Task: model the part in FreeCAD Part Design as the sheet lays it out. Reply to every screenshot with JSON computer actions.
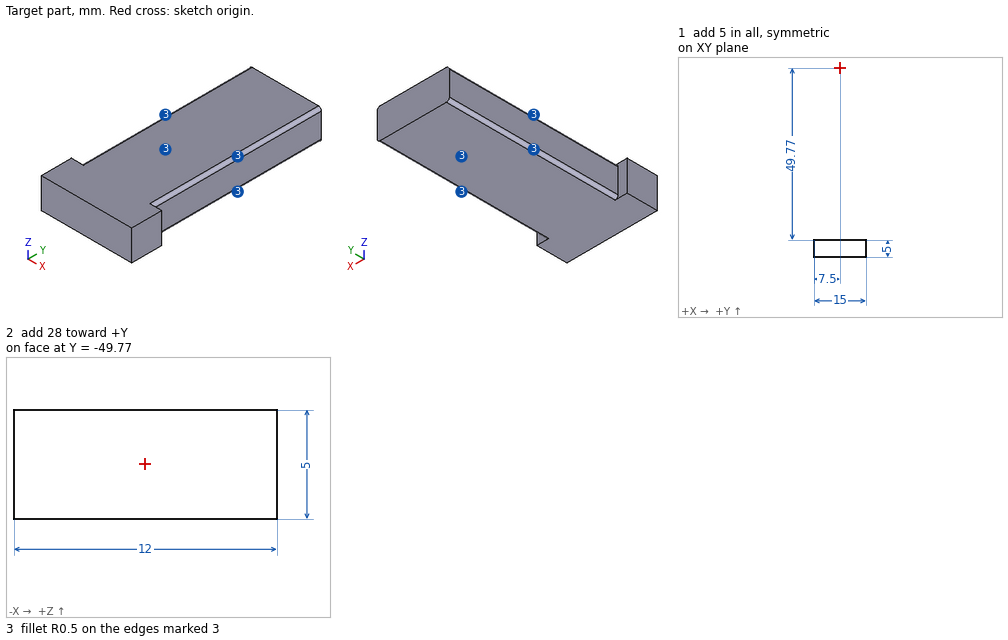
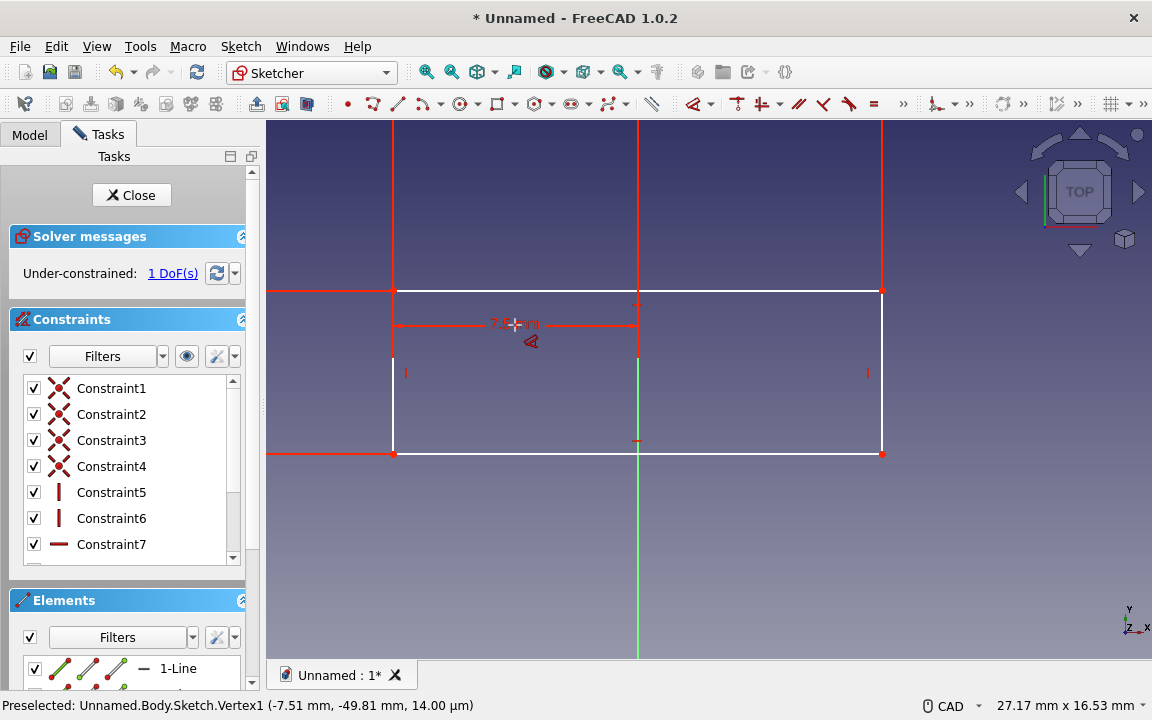
{"action": "left_click", "coordinate": [393, 291]}
{"action": "left_click", "coordinate": [359, 220]}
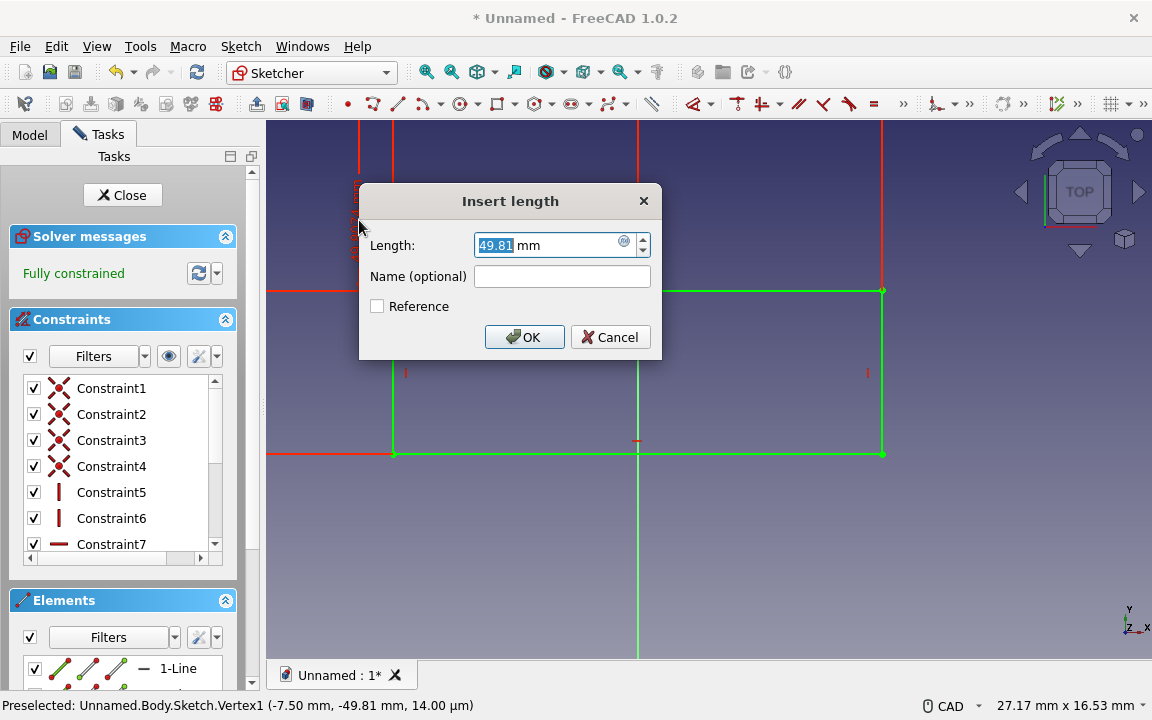
{"action": "type", "text": "49.77"}
{"action": "key", "text": "Return"}
{"action": "key", "text": "Escape"}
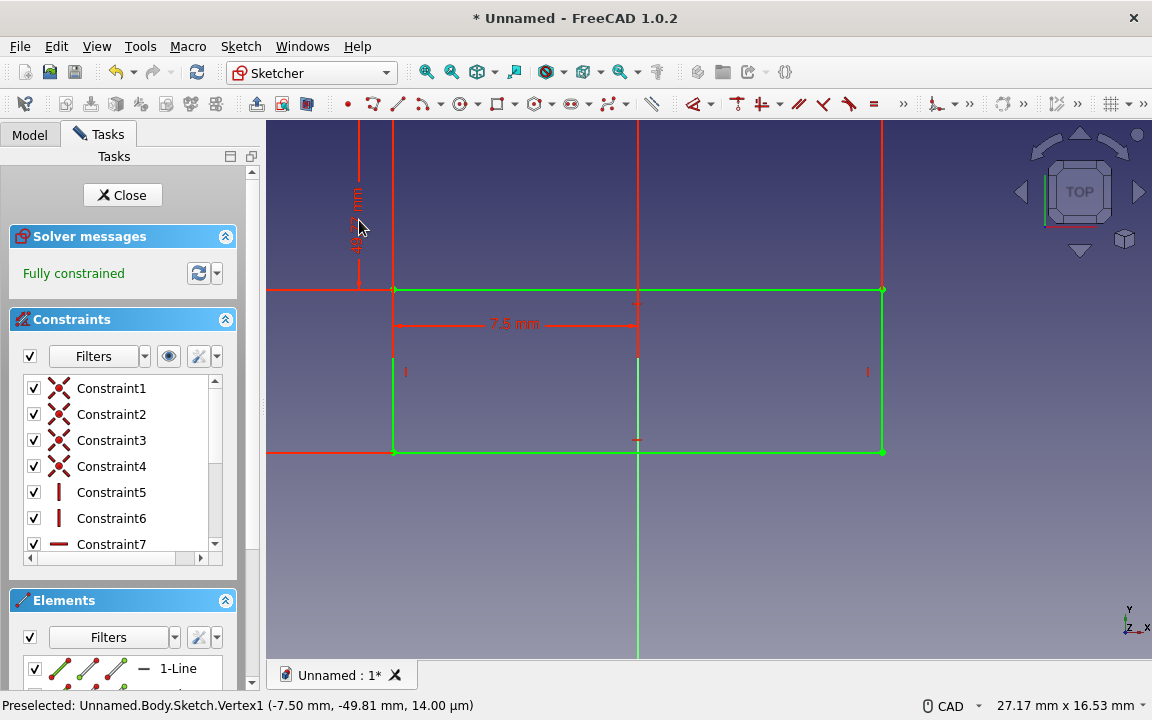
{"action": "left_click", "coordinate": [123, 195]}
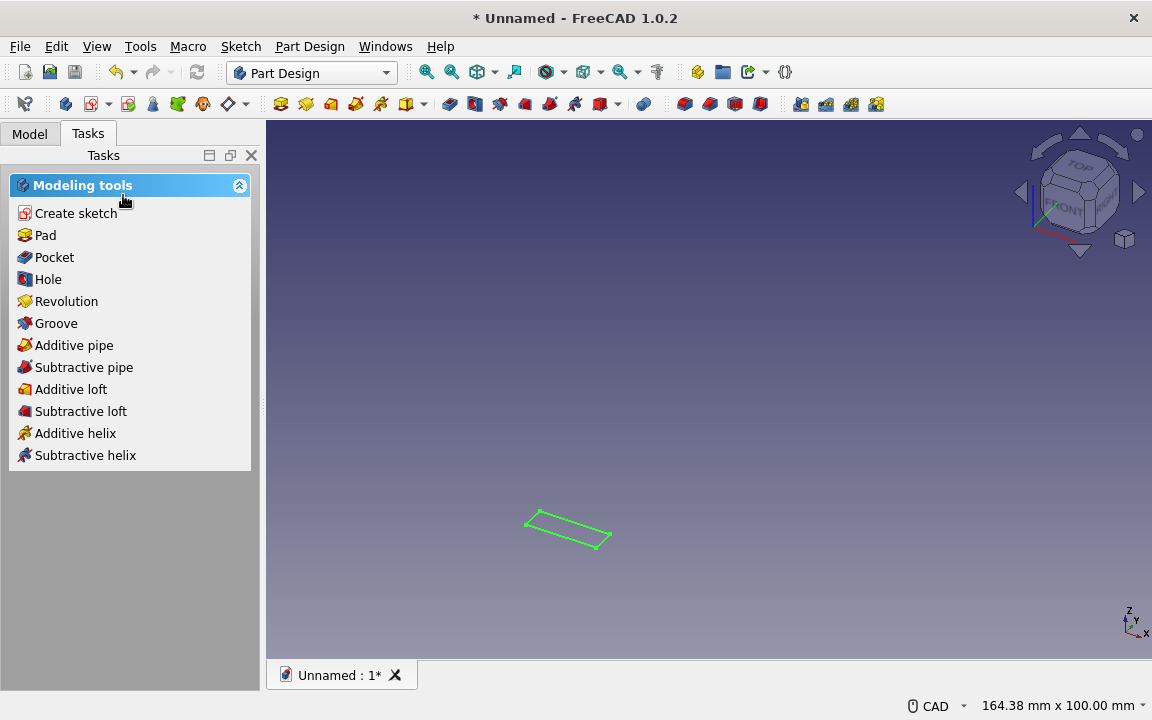
{"action": "left_click", "coordinate": [281, 104]}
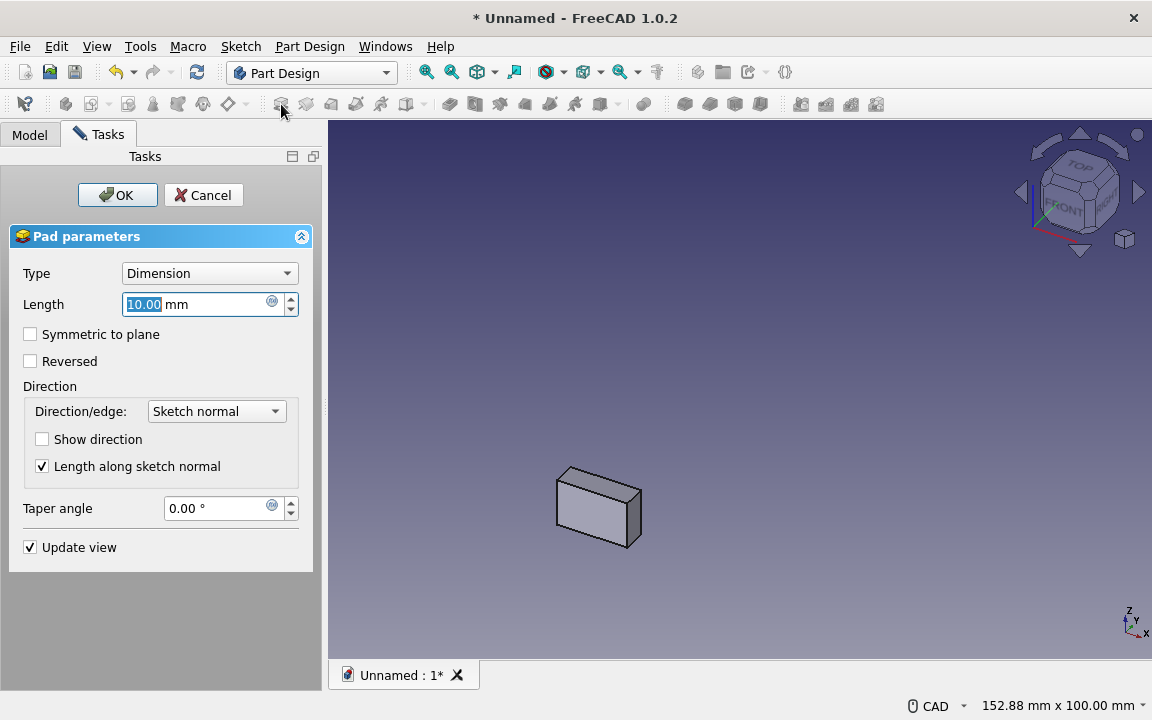
{"action": "type", "text": "5"}
{"action": "key", "text": "Tab"}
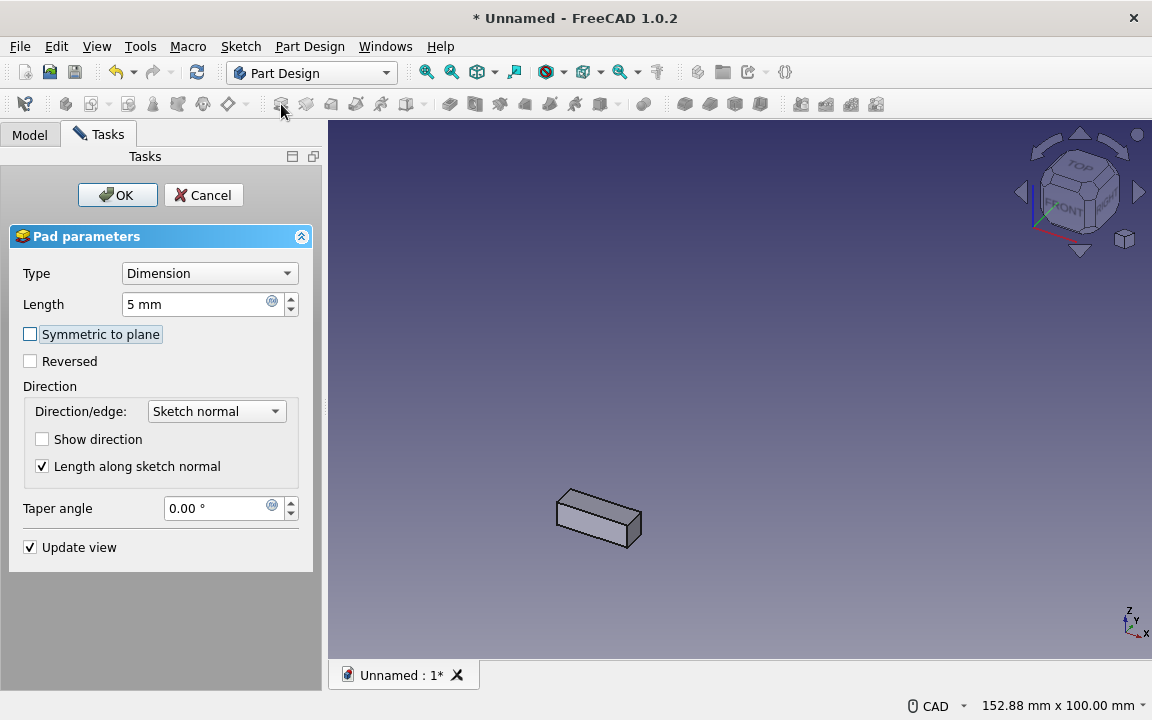
{"action": "left_click", "coordinate": [31, 334]}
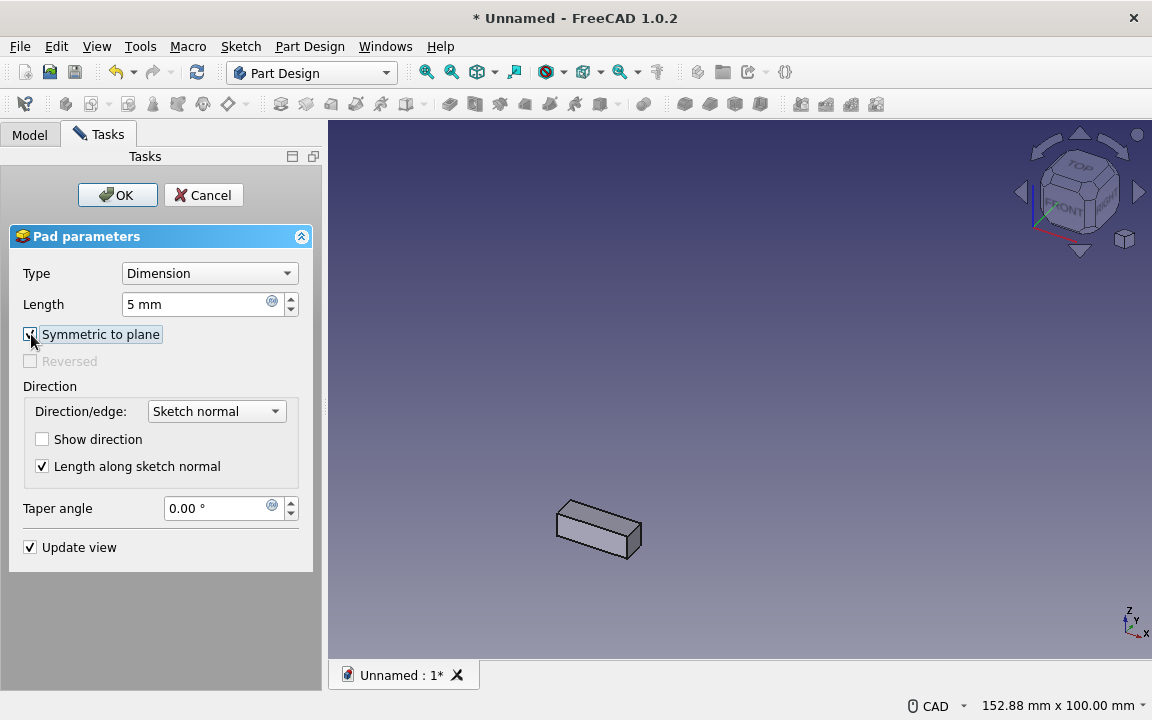
{"action": "left_click", "coordinate": [118, 195]}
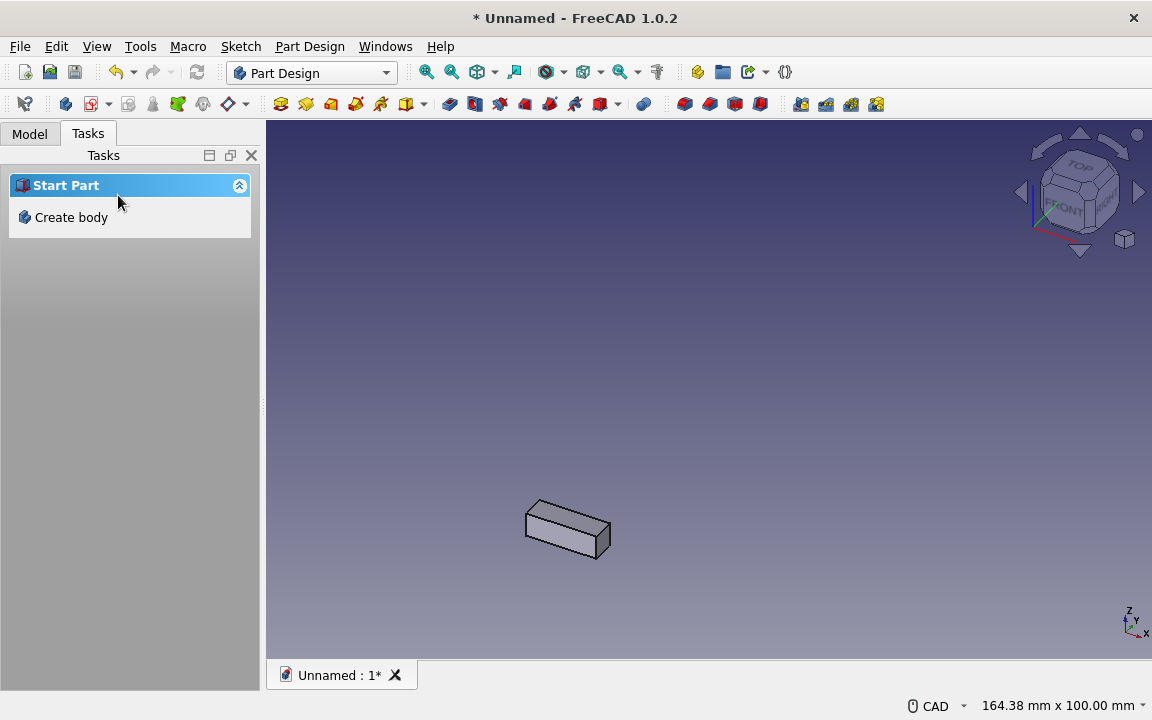
{"action": "key", "text": "v f"}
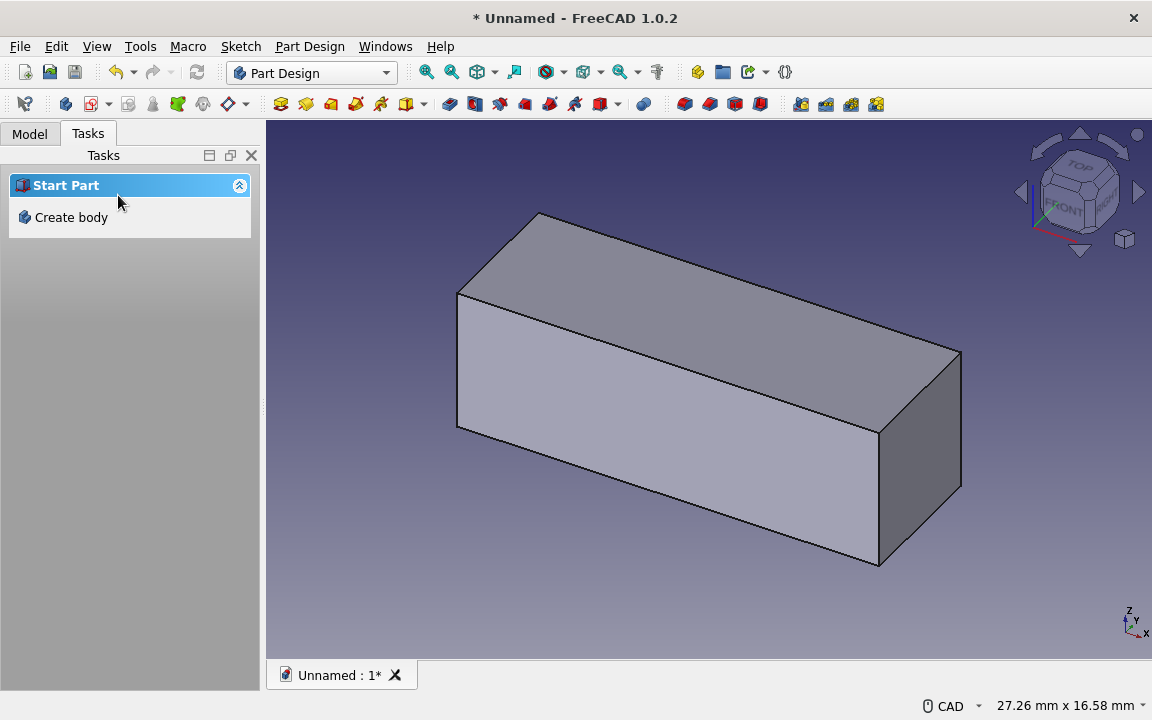
{"action": "key", "text": "4"}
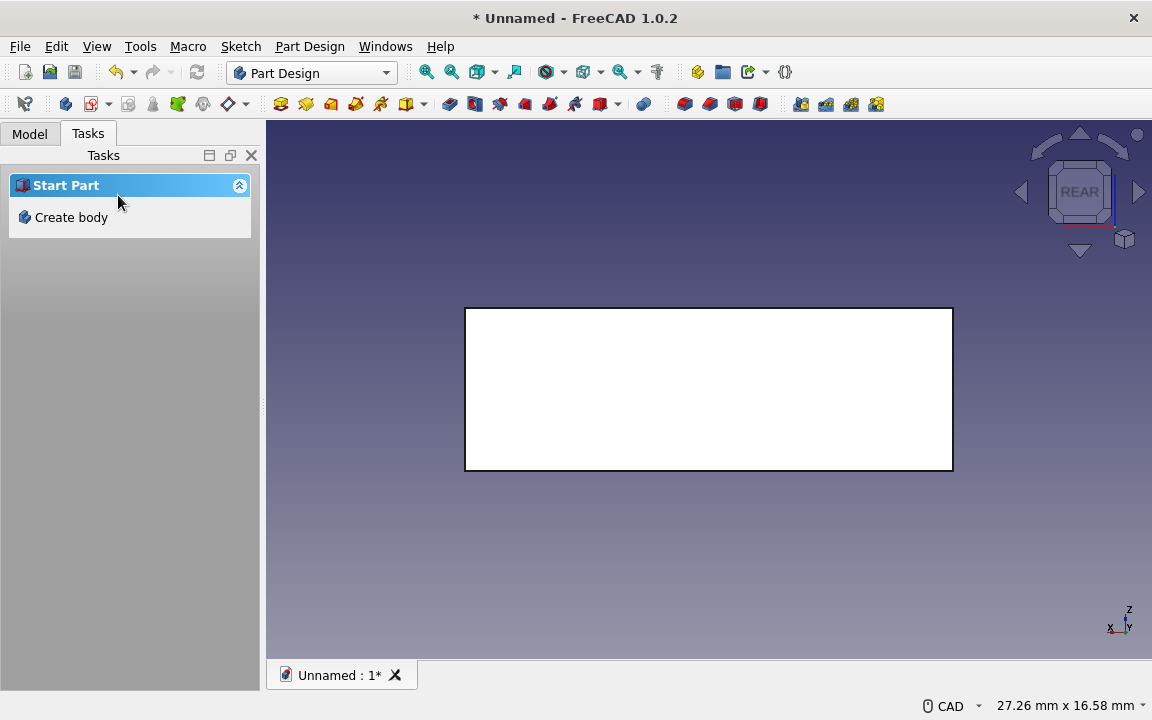
{"action": "left_click", "coordinate": [570, 389]}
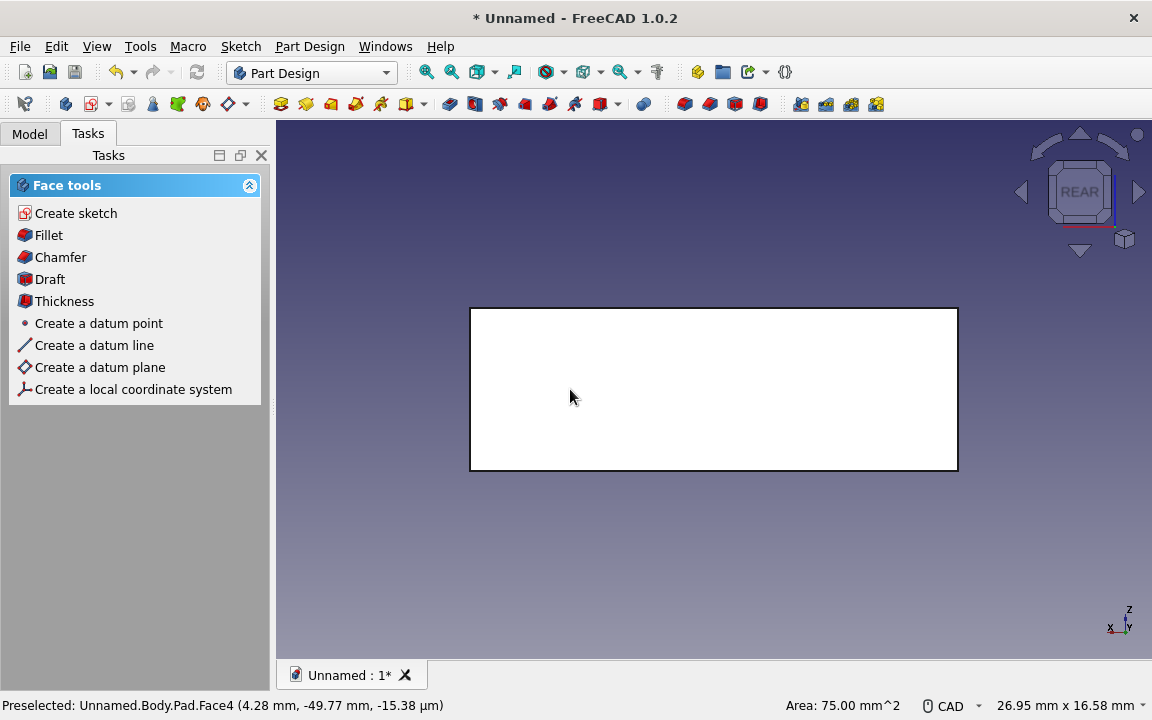
{"action": "left_click", "coordinate": [90, 104]}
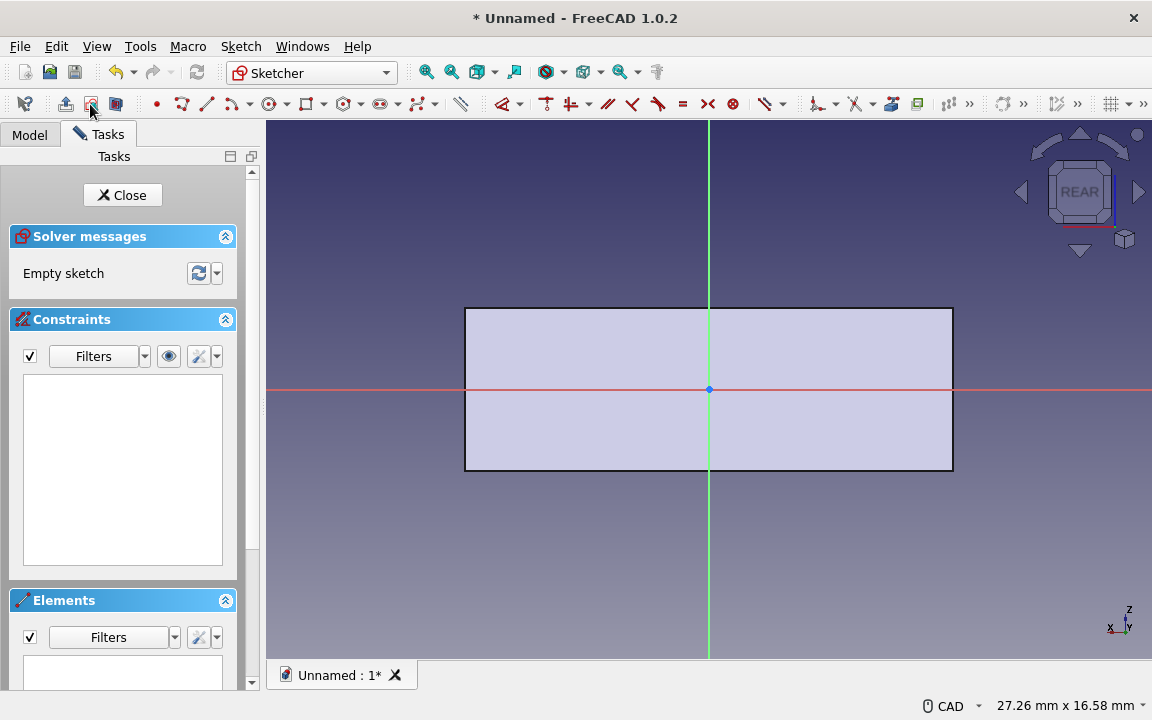
{"action": "key", "text": "g v"}